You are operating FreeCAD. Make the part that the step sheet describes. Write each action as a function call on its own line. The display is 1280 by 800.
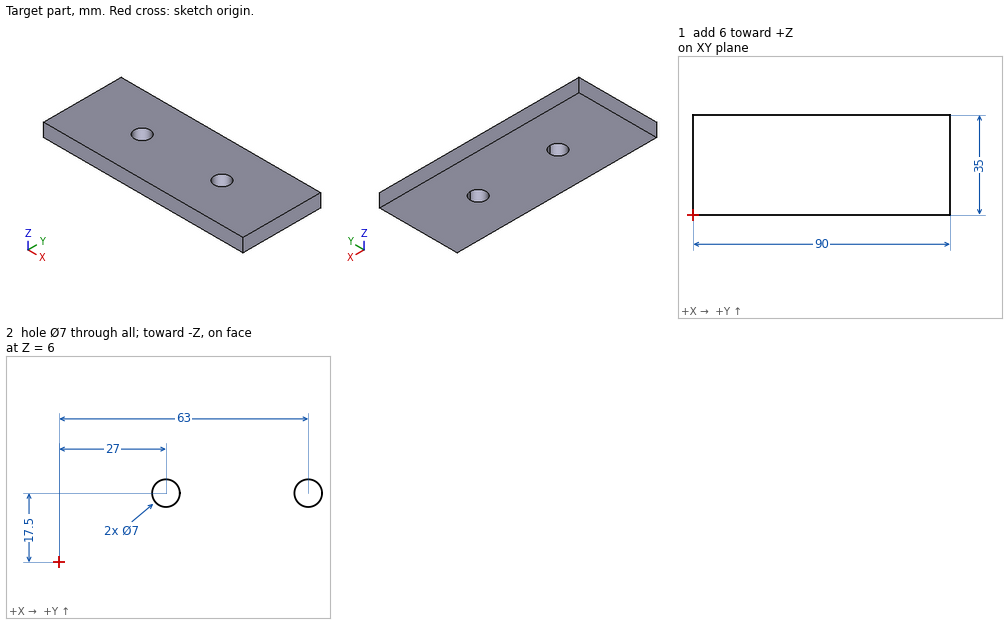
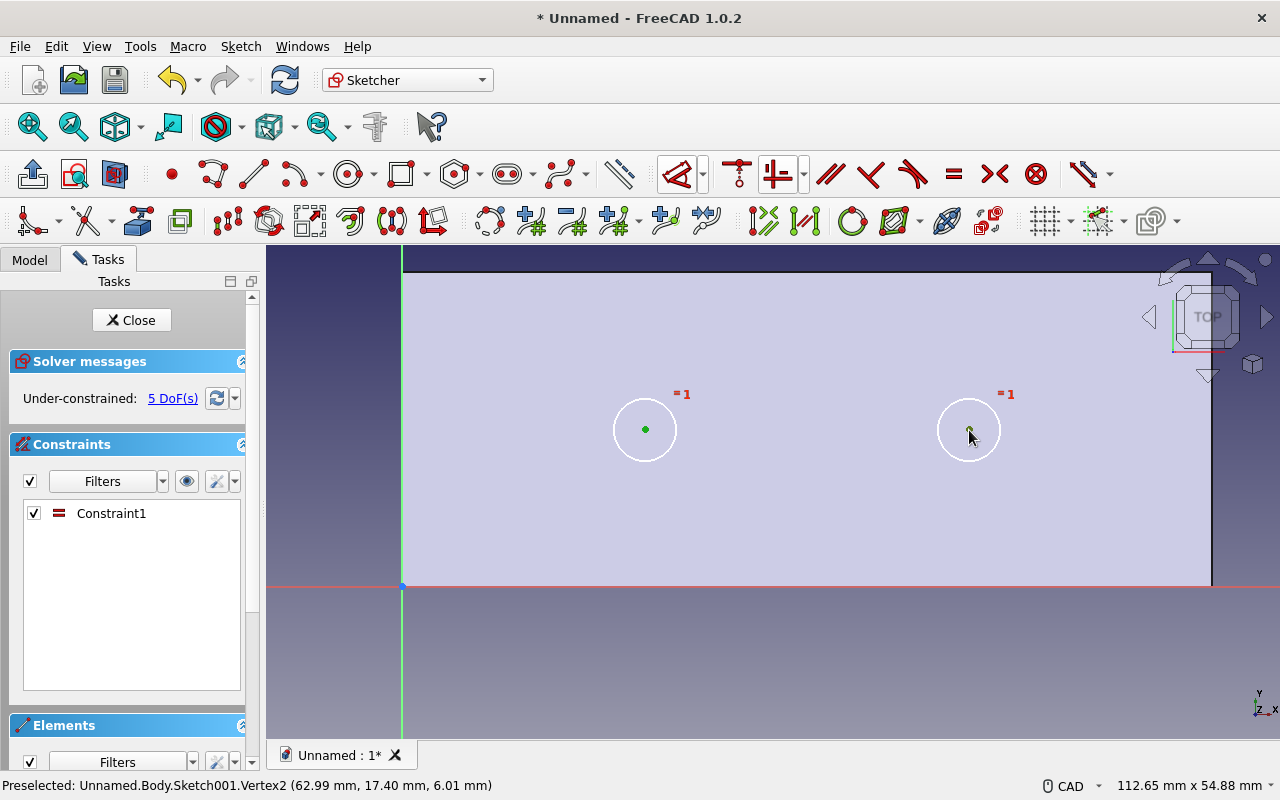
key(h)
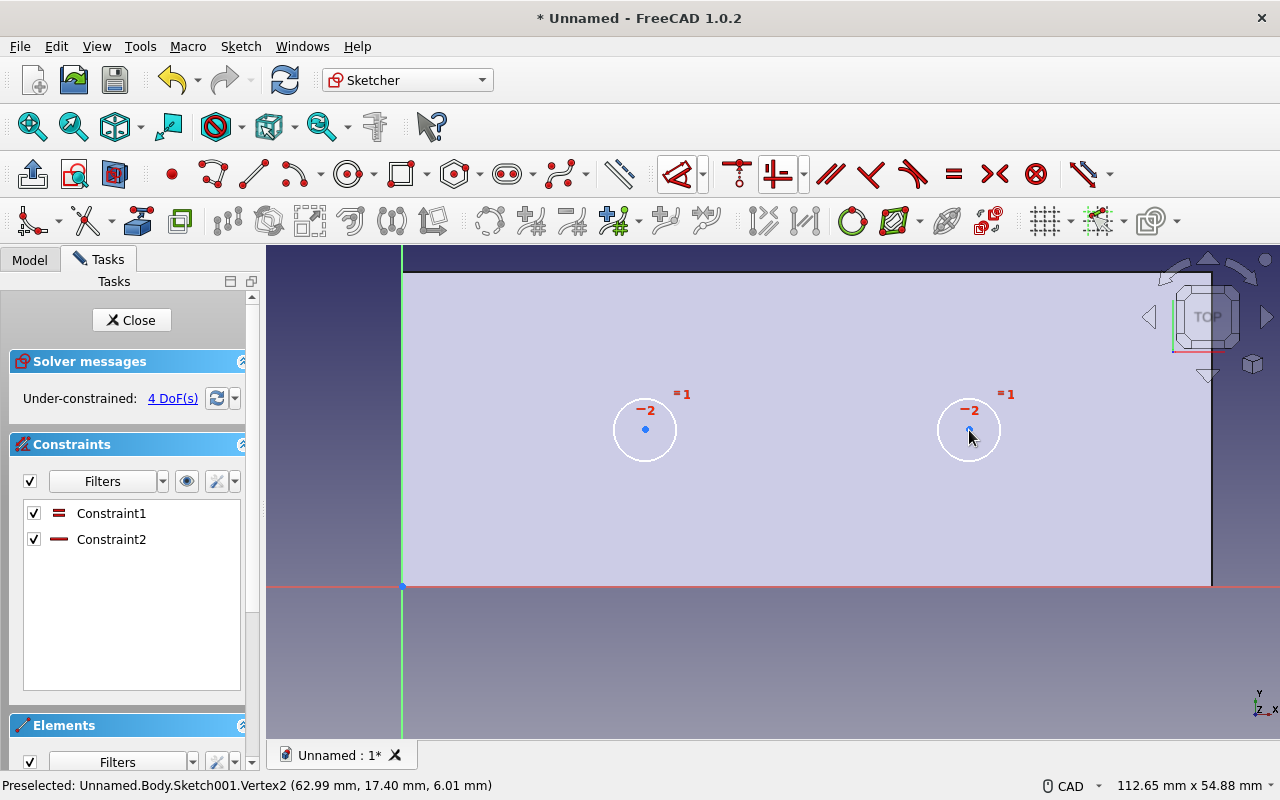
click(667, 408)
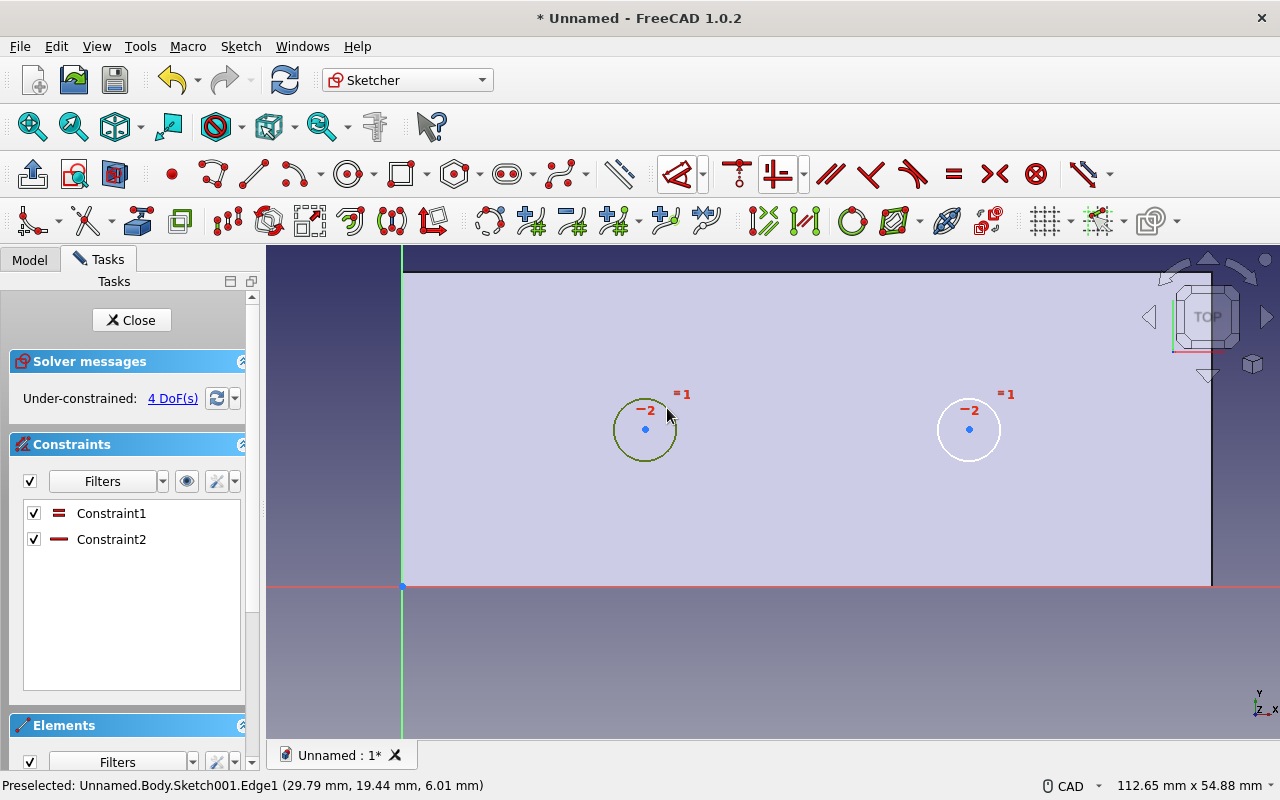
key(k)
key(o)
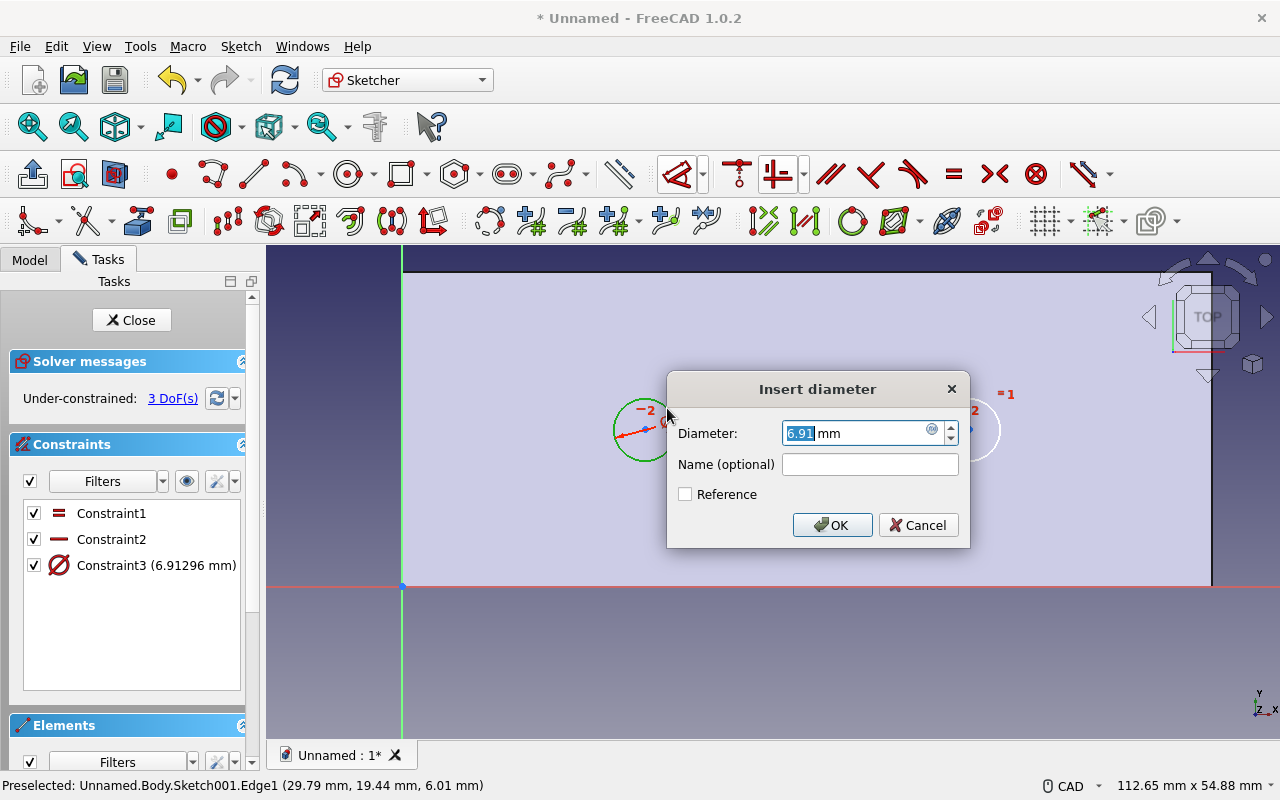
text(7)
key(Return)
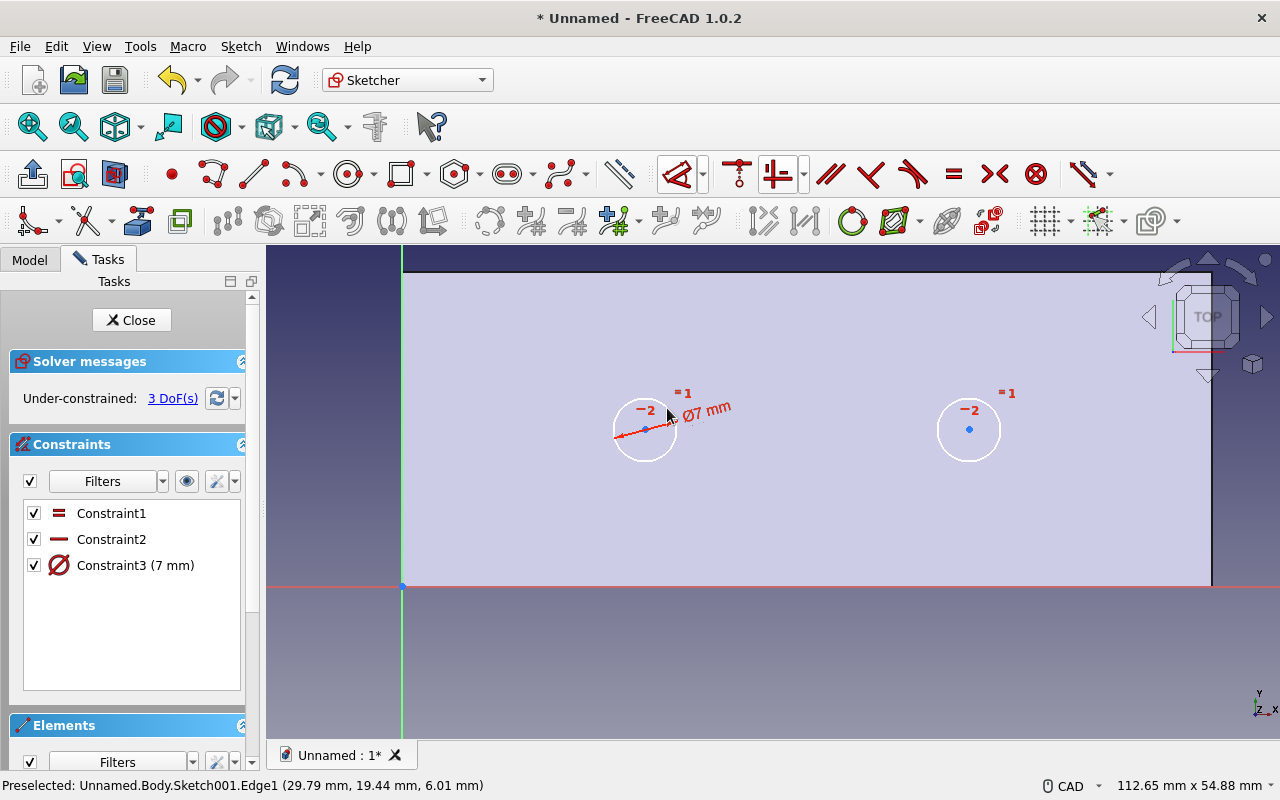
click(645, 430)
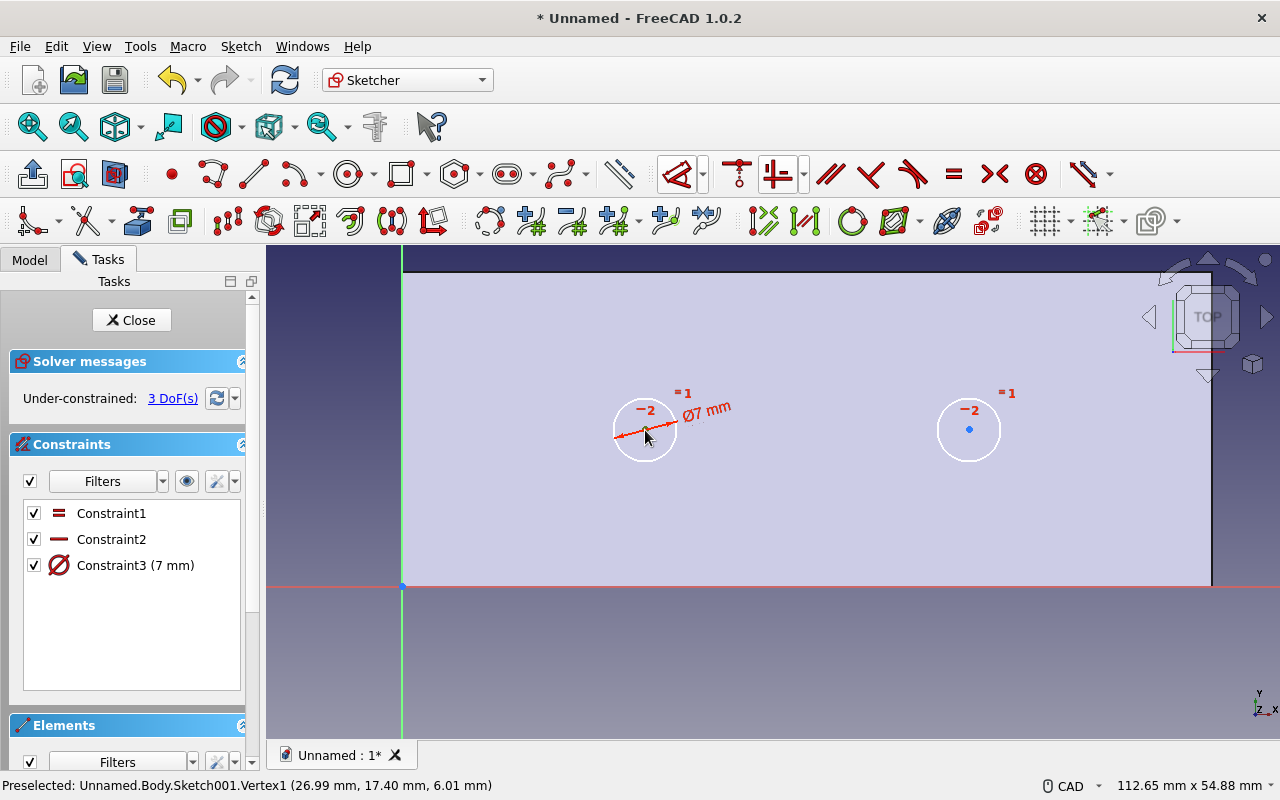
key(l)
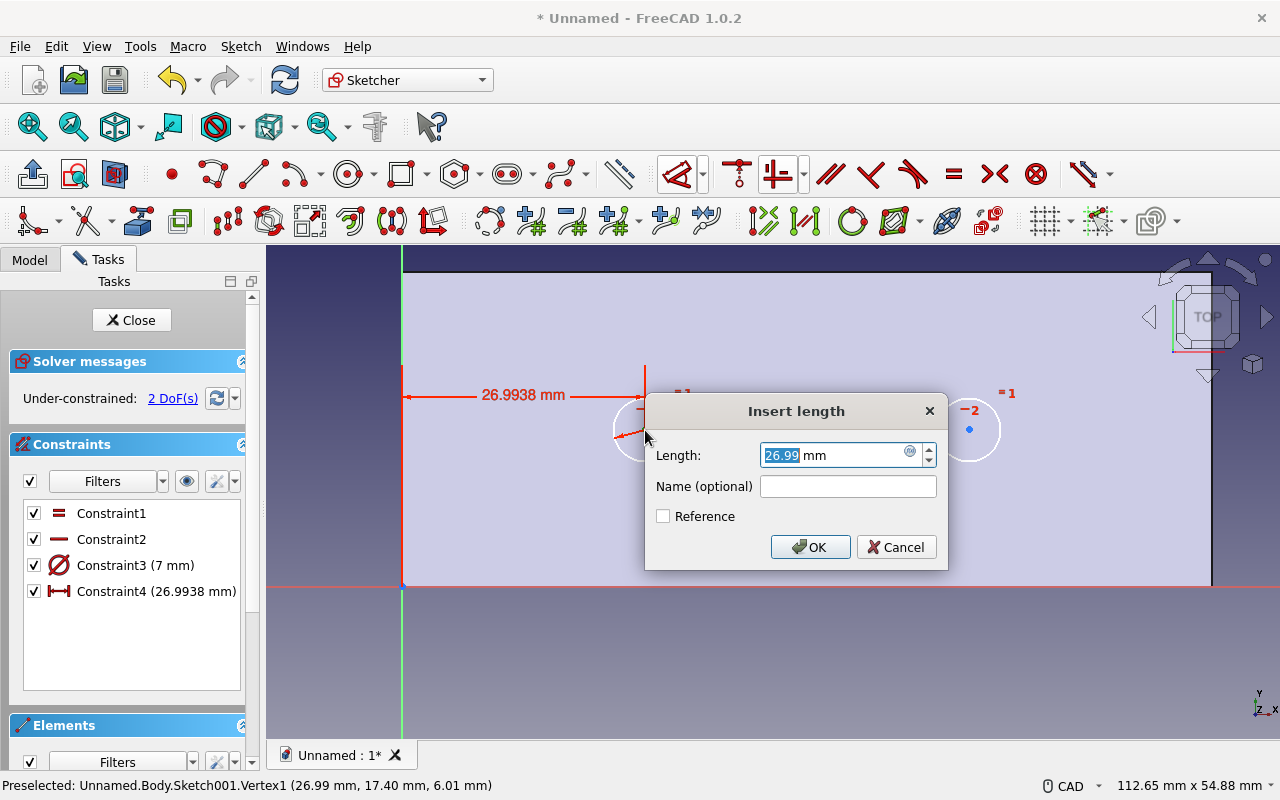
text(27)
key(Return)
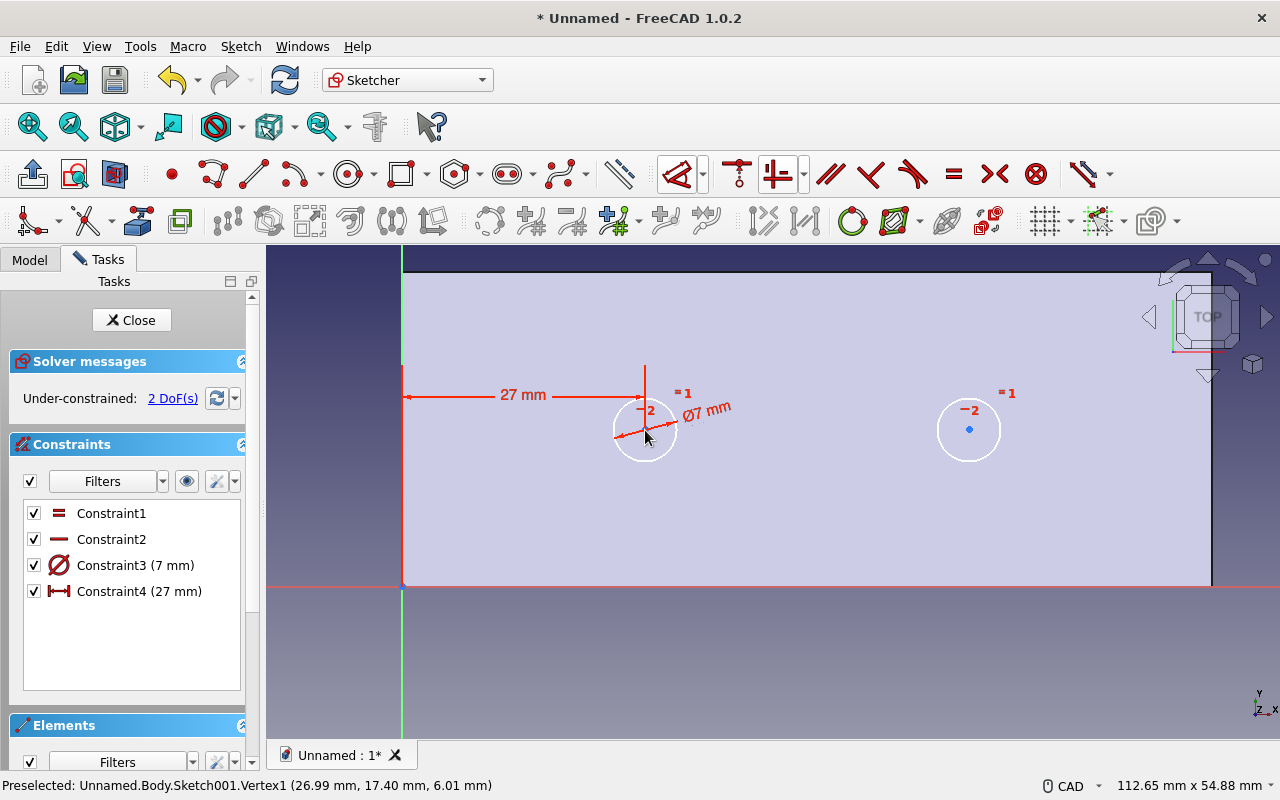
click(969, 430)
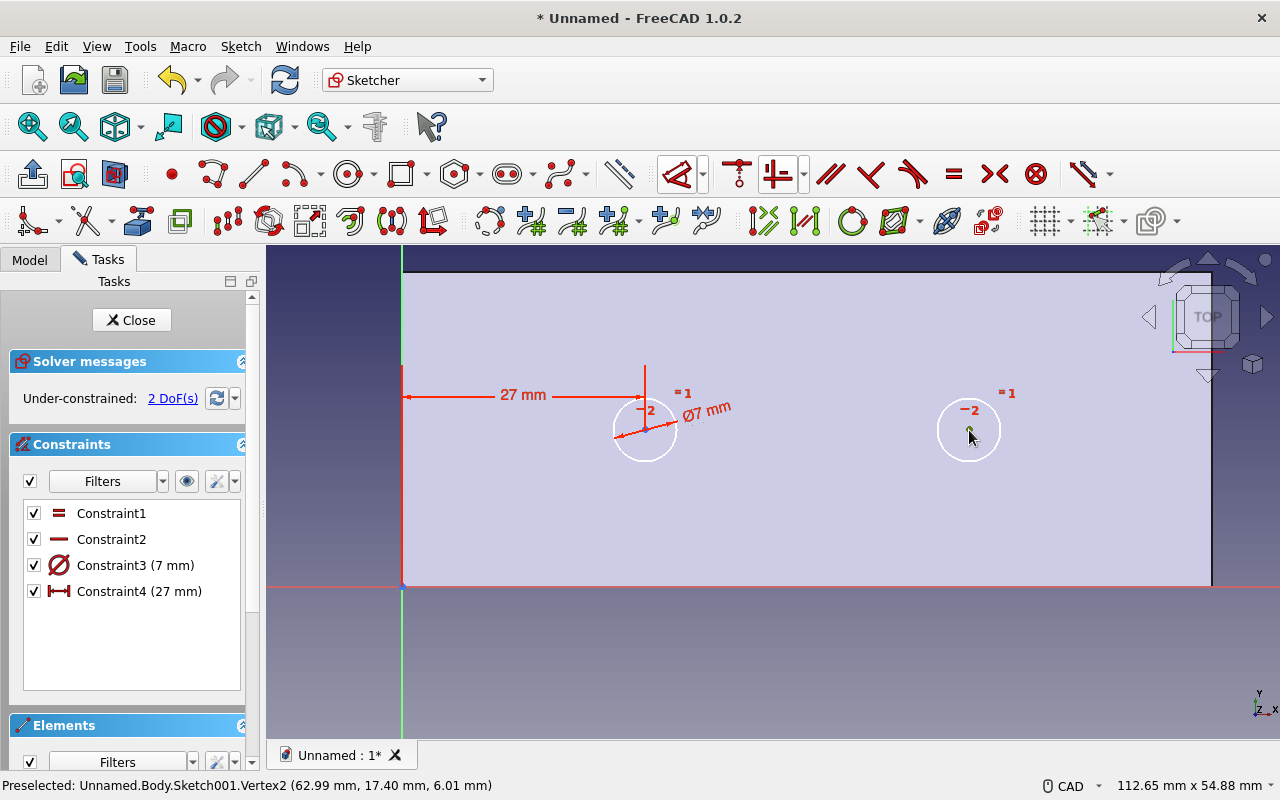
key(l)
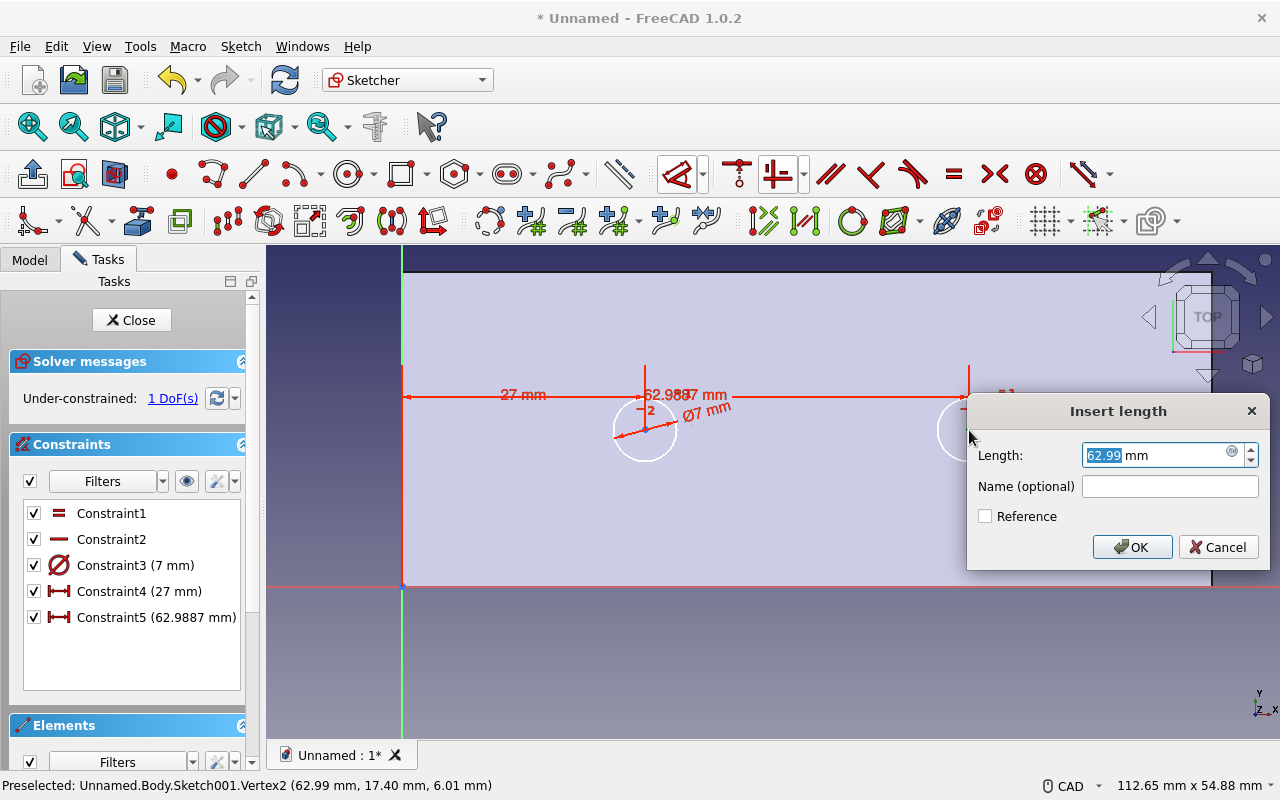
text(63)
key(Return)